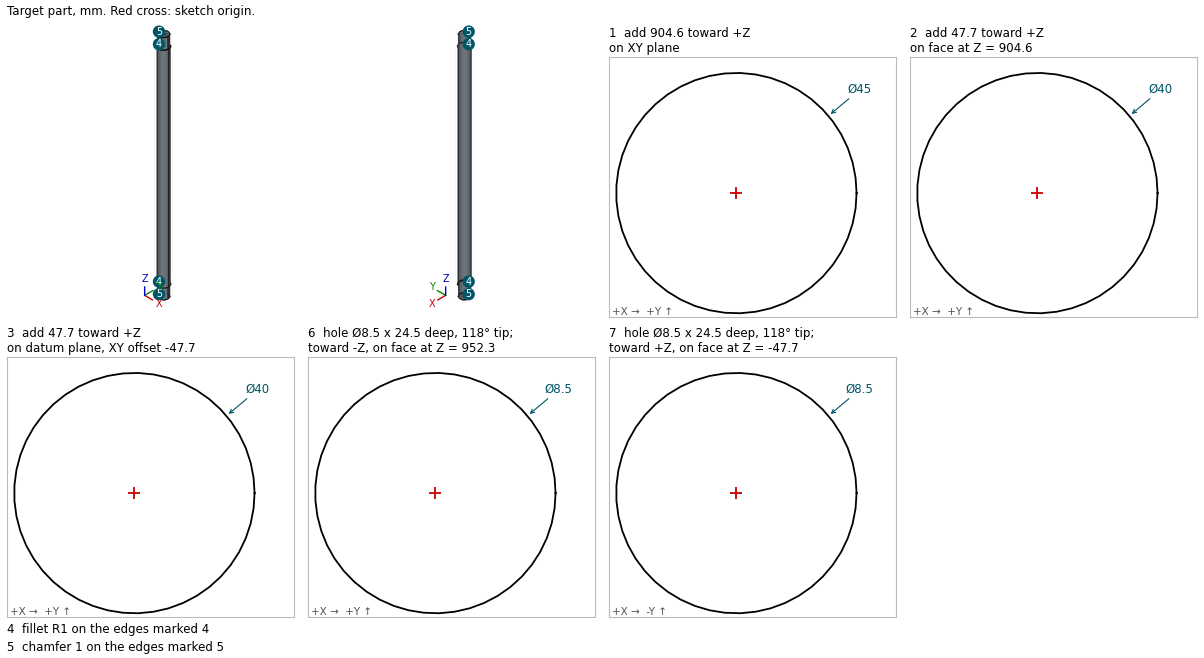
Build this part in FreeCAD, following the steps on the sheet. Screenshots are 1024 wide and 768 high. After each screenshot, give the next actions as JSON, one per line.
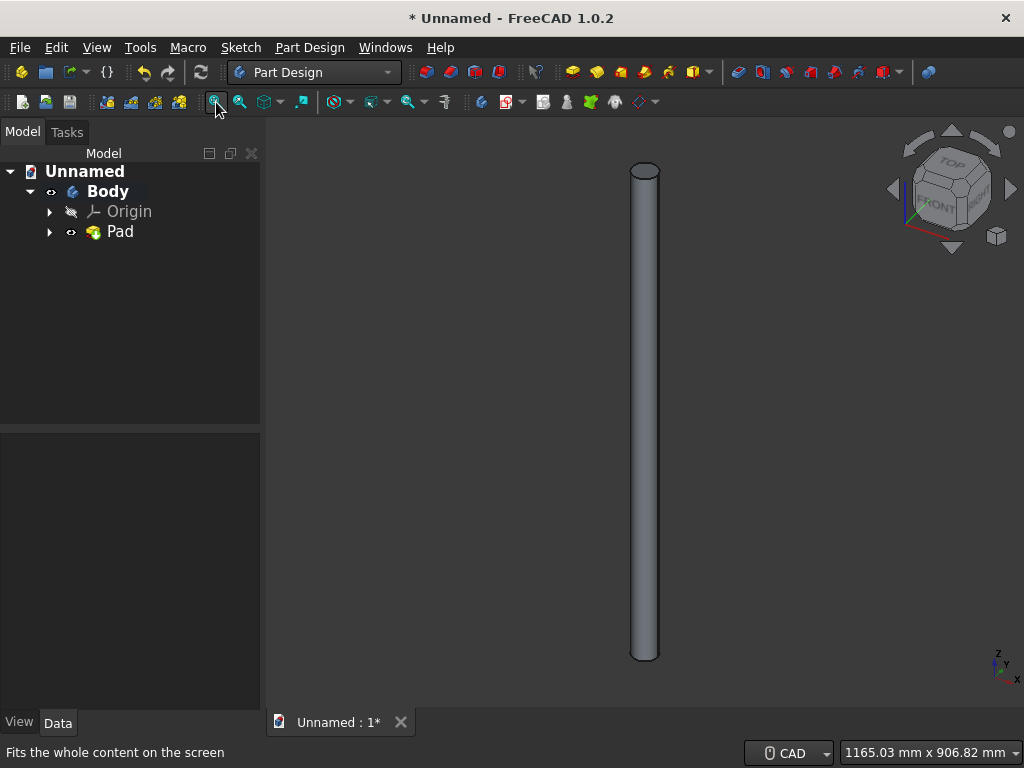
{"action": "left_click", "coordinate": [645, 170]}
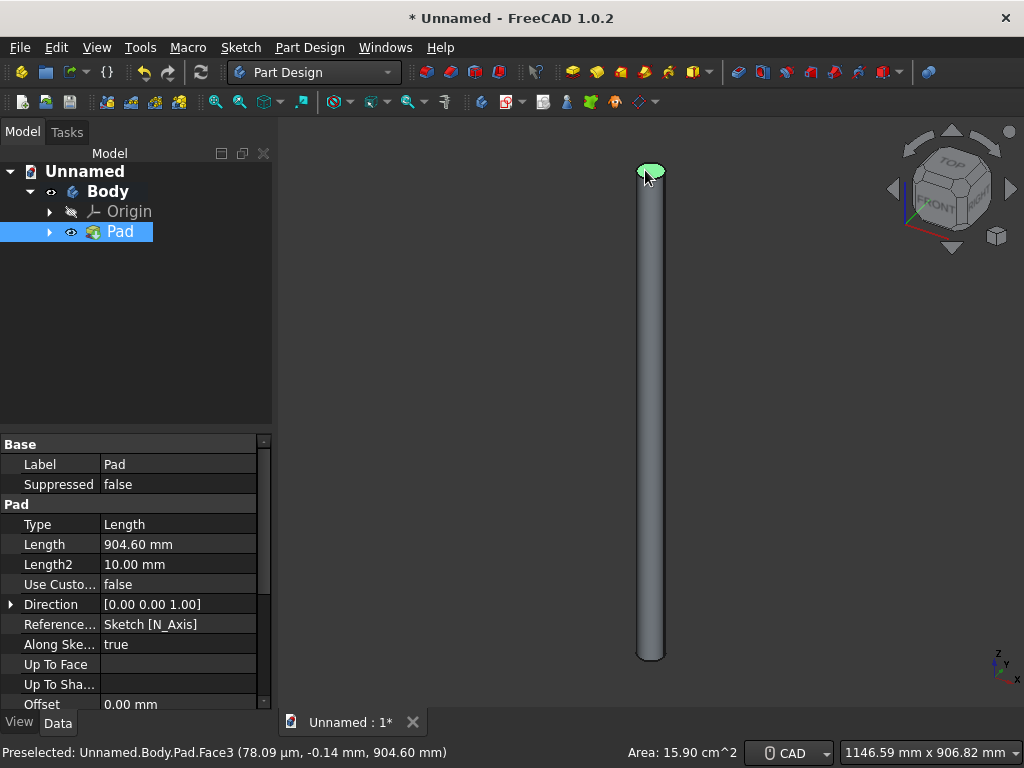
{"action": "left_click", "coordinate": [506, 102]}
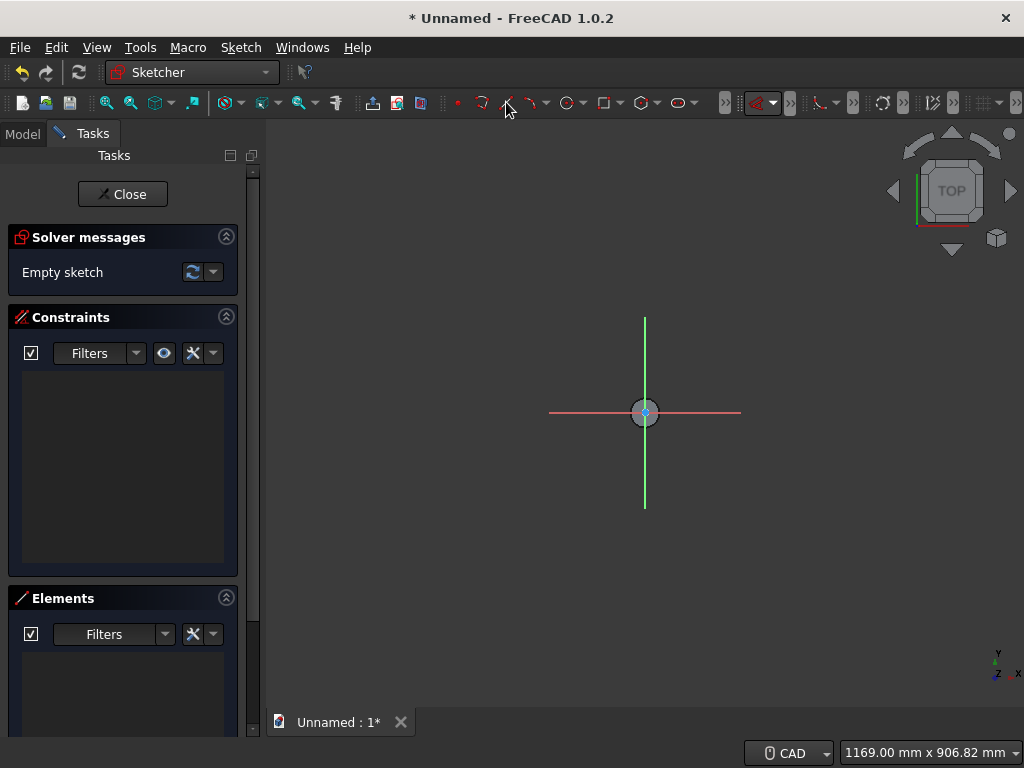
{"action": "scroll", "coordinate": [650, 413], "scroll_direction": "up", "scroll_amount": 13}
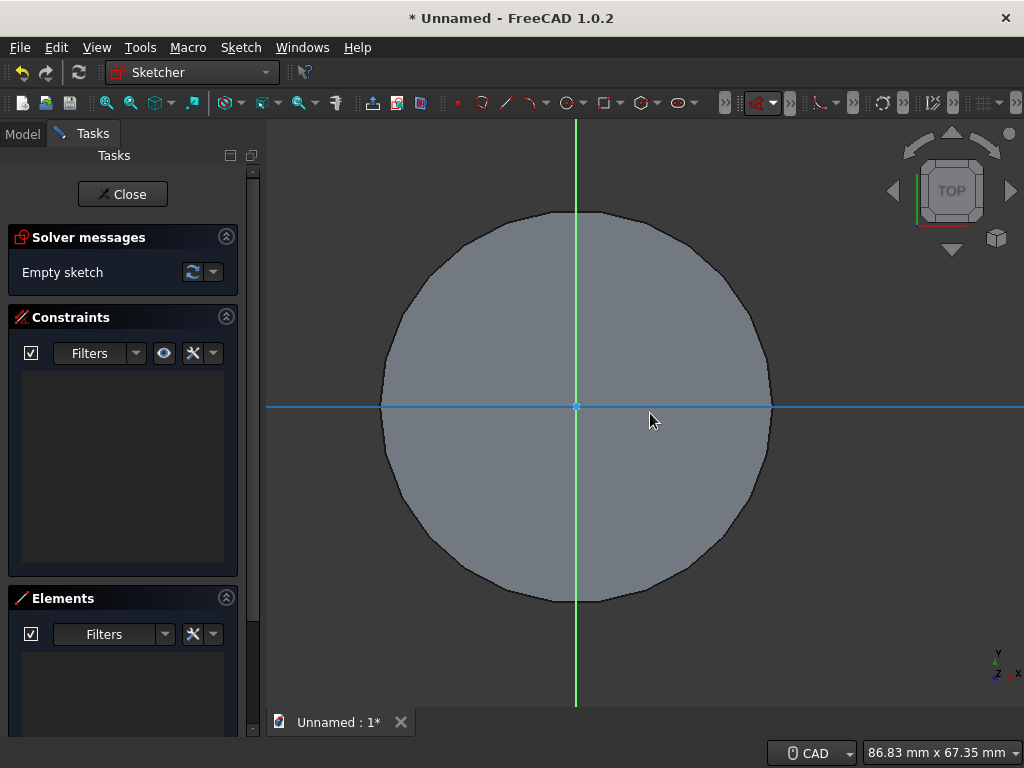
{"action": "left_click", "coordinate": [568, 104]}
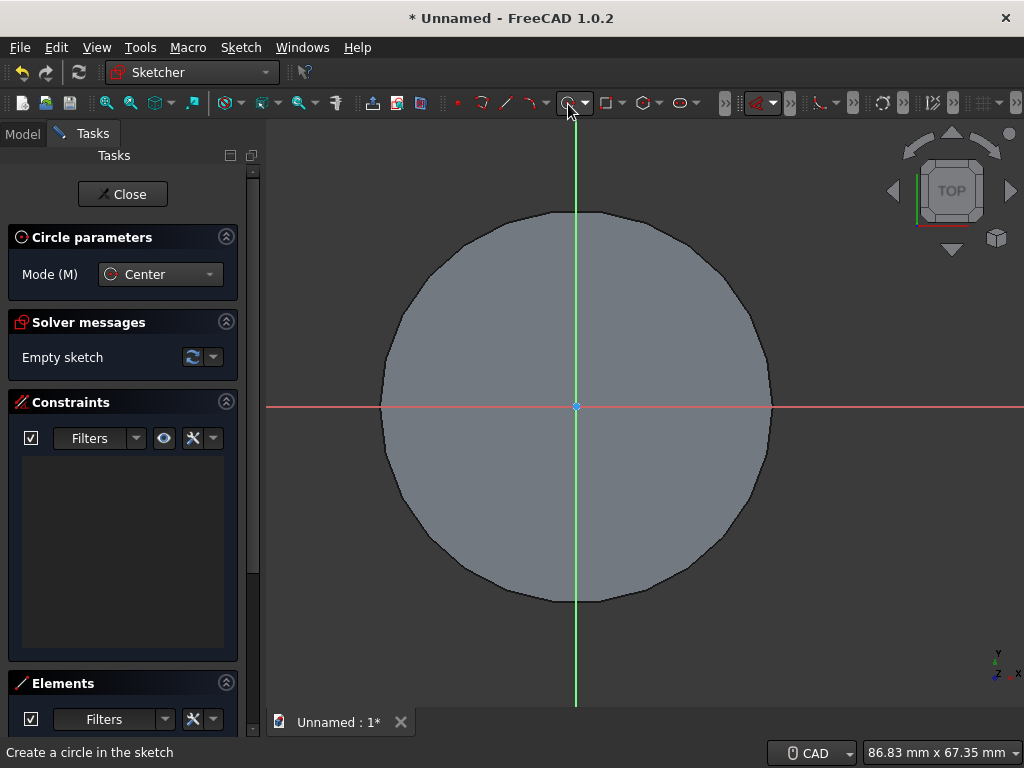
{"action": "left_click", "coordinate": [576, 407]}
{"action": "mouse_move", "coordinate": [700, 283]}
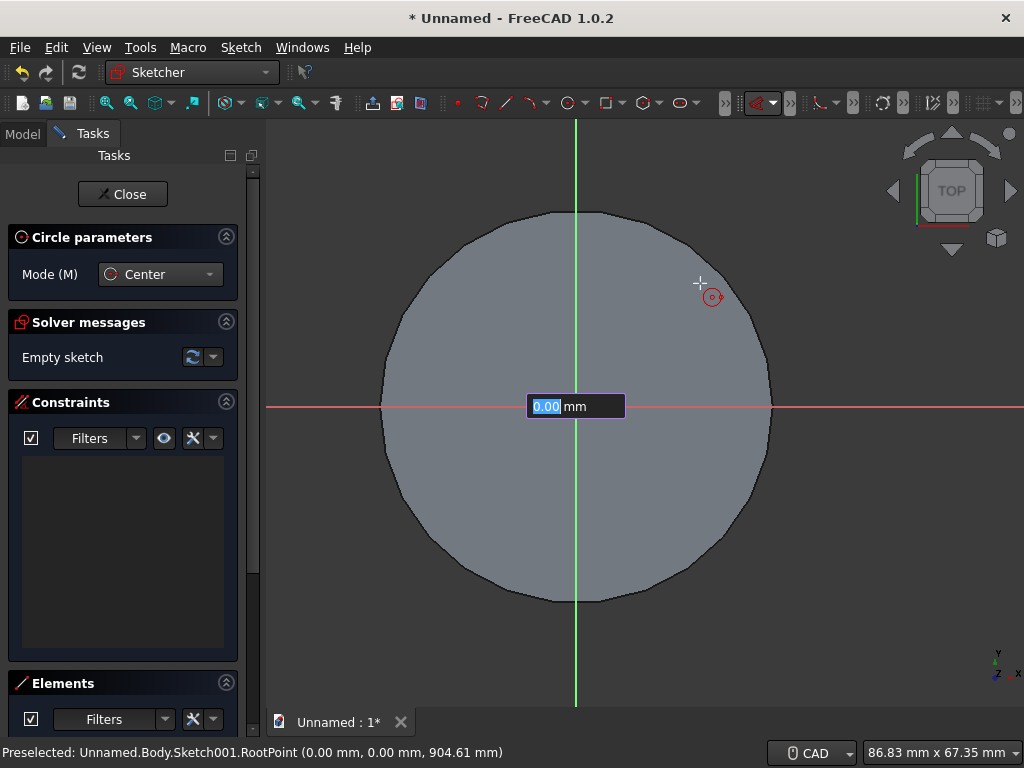
{"action": "type", "text": "40"}
{"action": "key", "text": "Return"}
{"action": "key", "text": "Escape"}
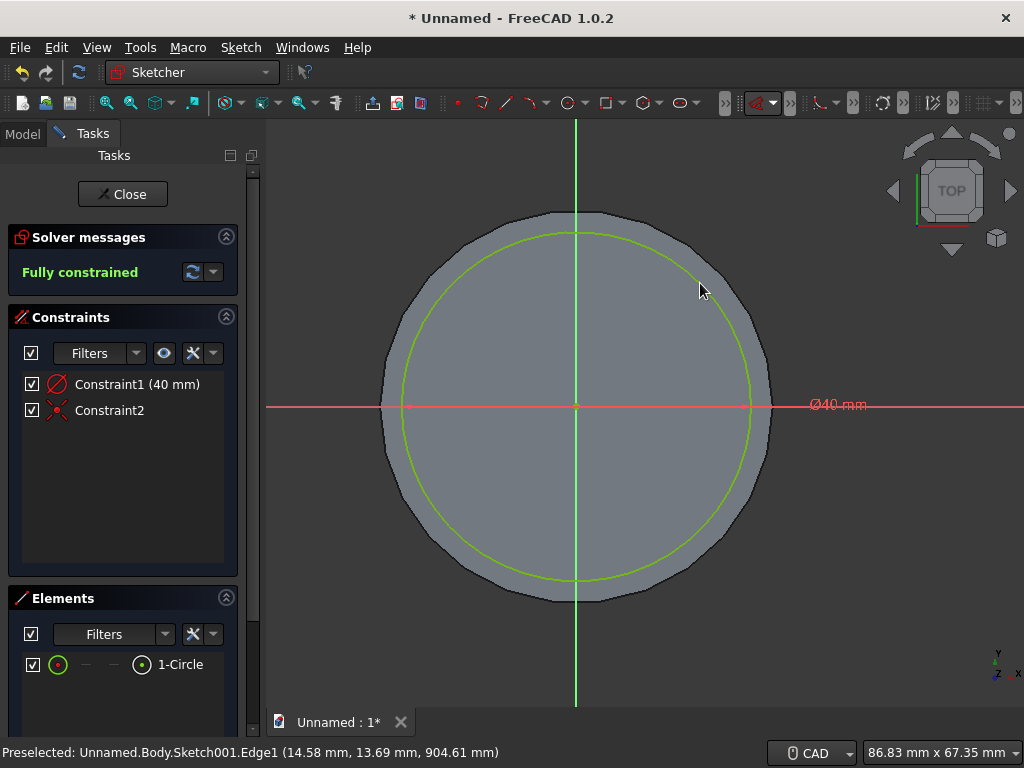
{"action": "left_click", "coordinate": [123, 194]}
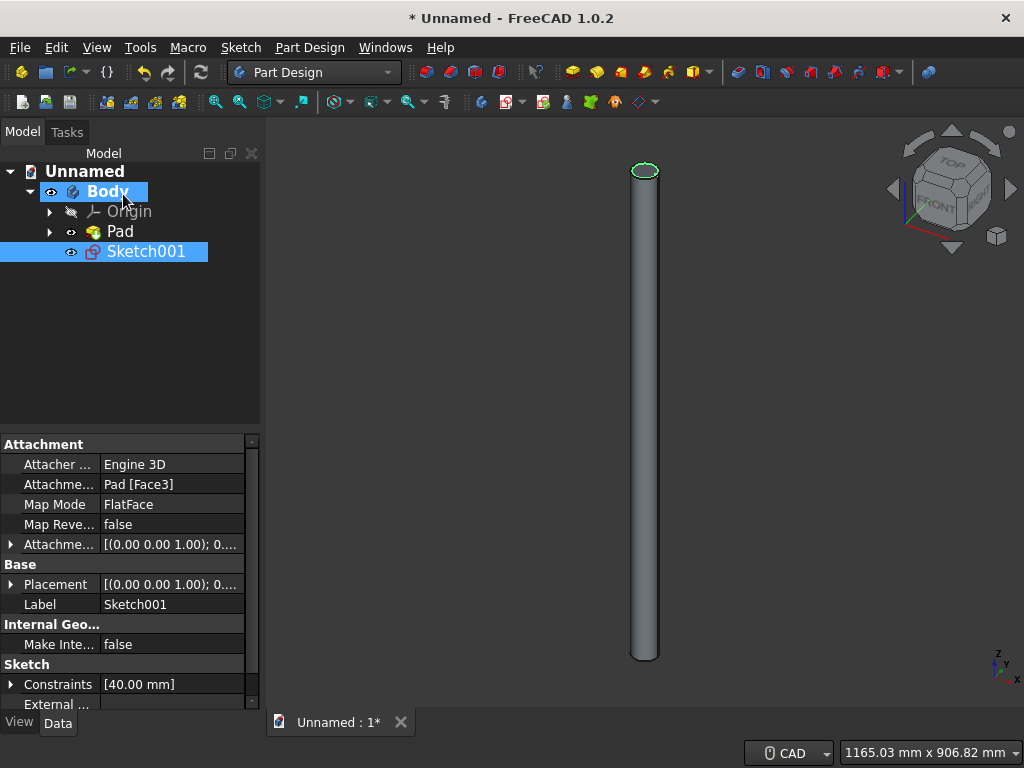
{"action": "left_click", "coordinate": [574, 72]}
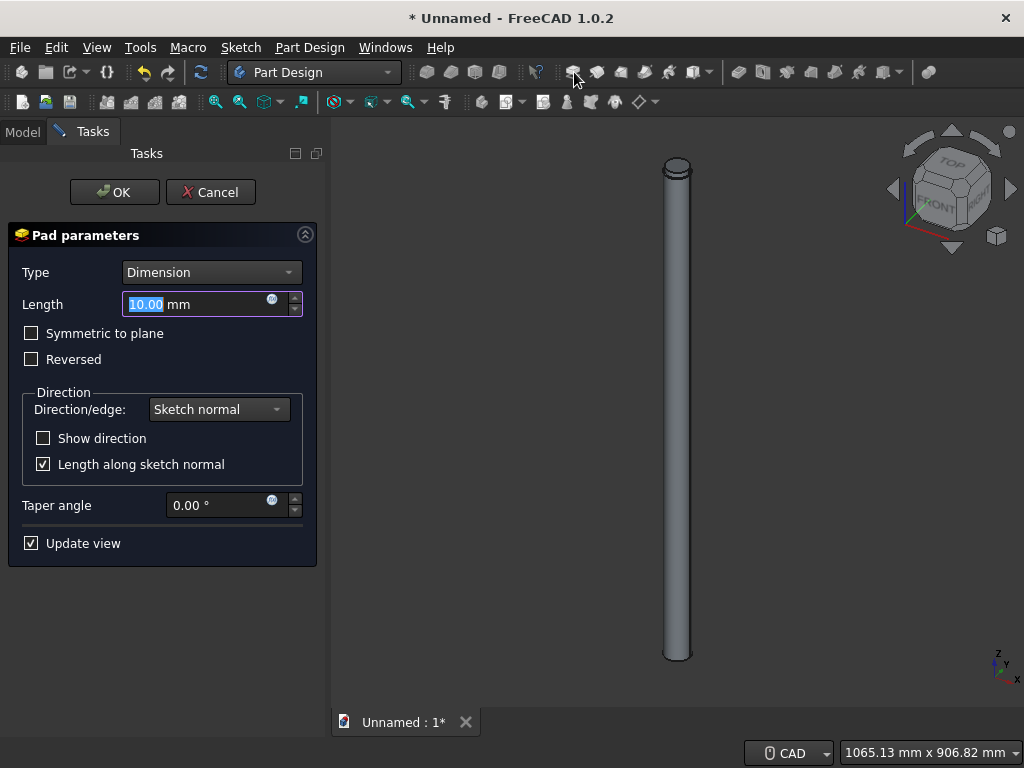
{"action": "type", "text": "47.7"}
{"action": "key", "text": "Tab"}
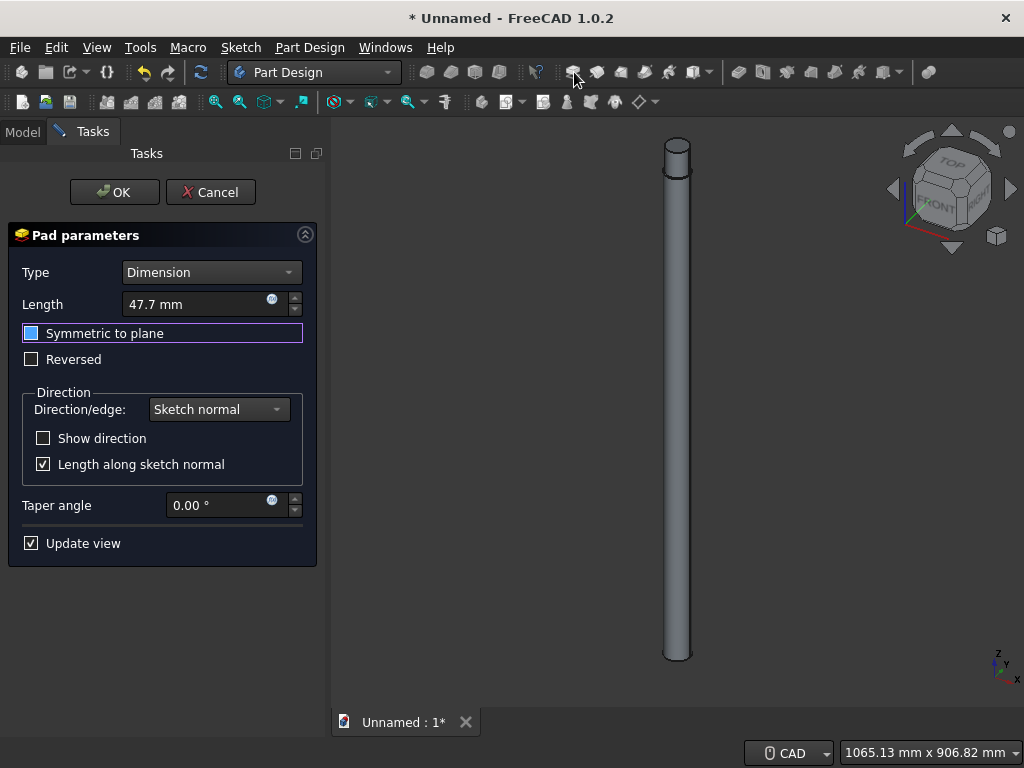
{"action": "left_click", "coordinate": [115, 192]}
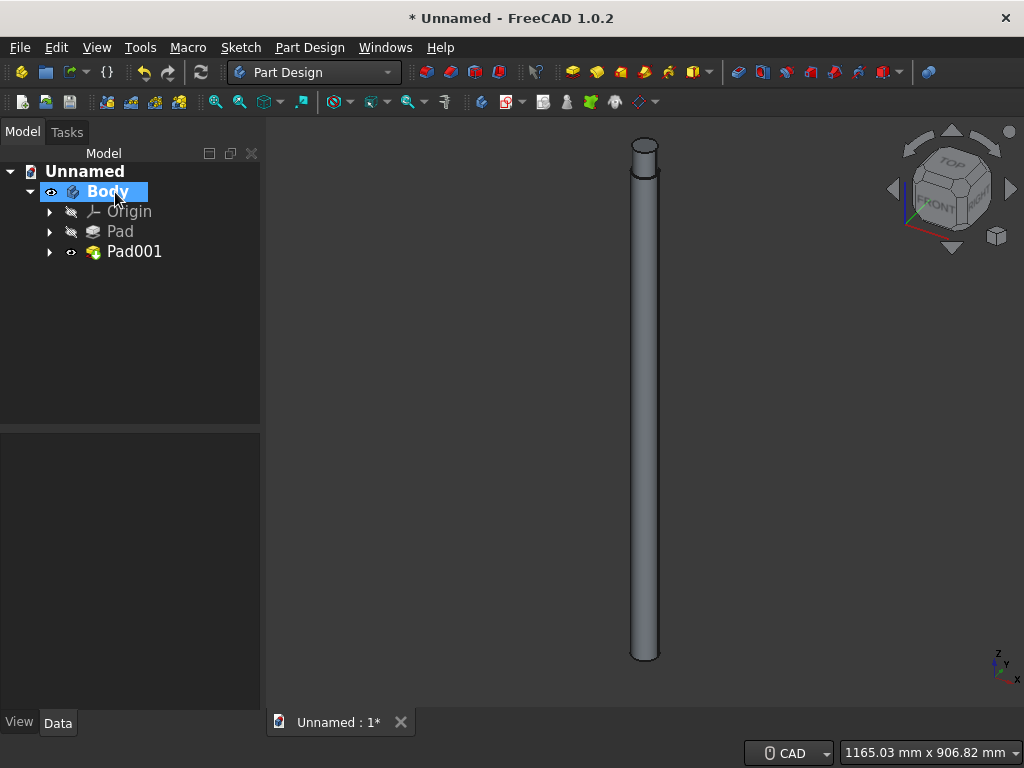
{"action": "left_click", "coordinate": [50, 212]}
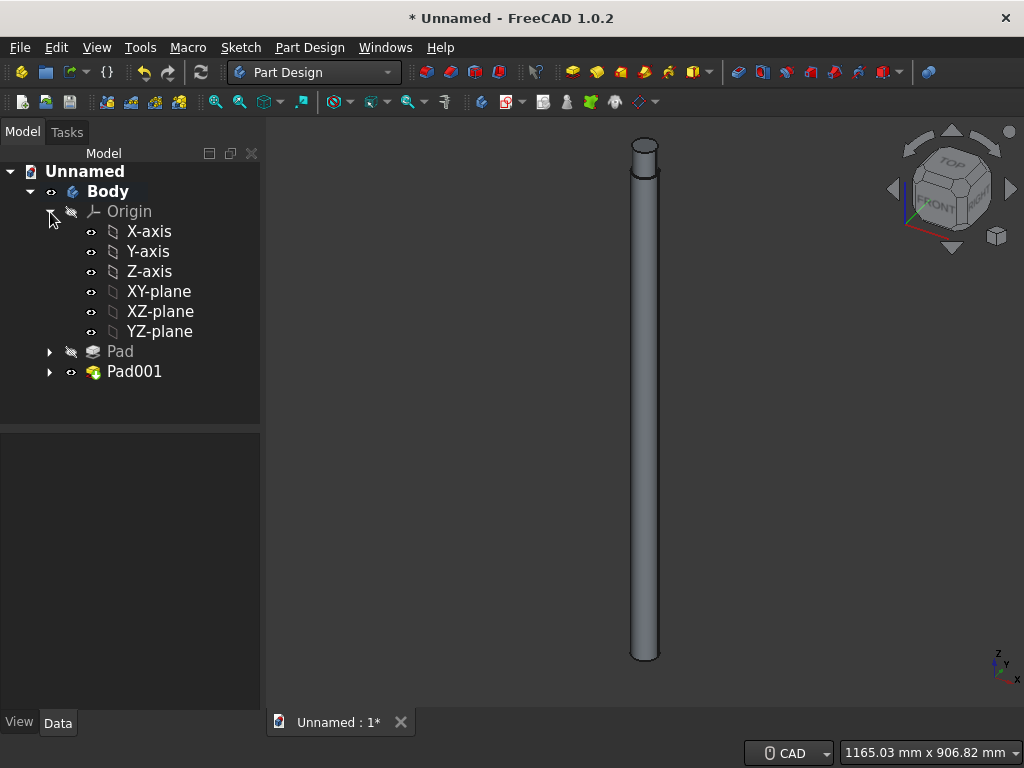
{"action": "left_click", "coordinate": [136, 292]}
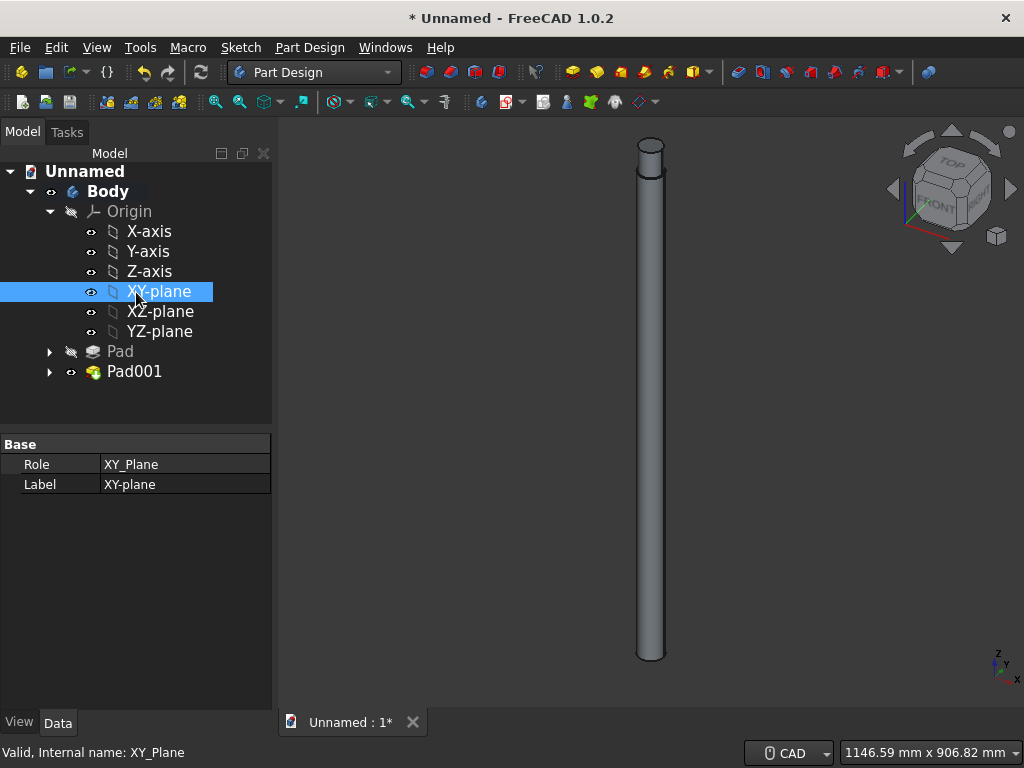
{"action": "left_click", "coordinate": [640, 102]}